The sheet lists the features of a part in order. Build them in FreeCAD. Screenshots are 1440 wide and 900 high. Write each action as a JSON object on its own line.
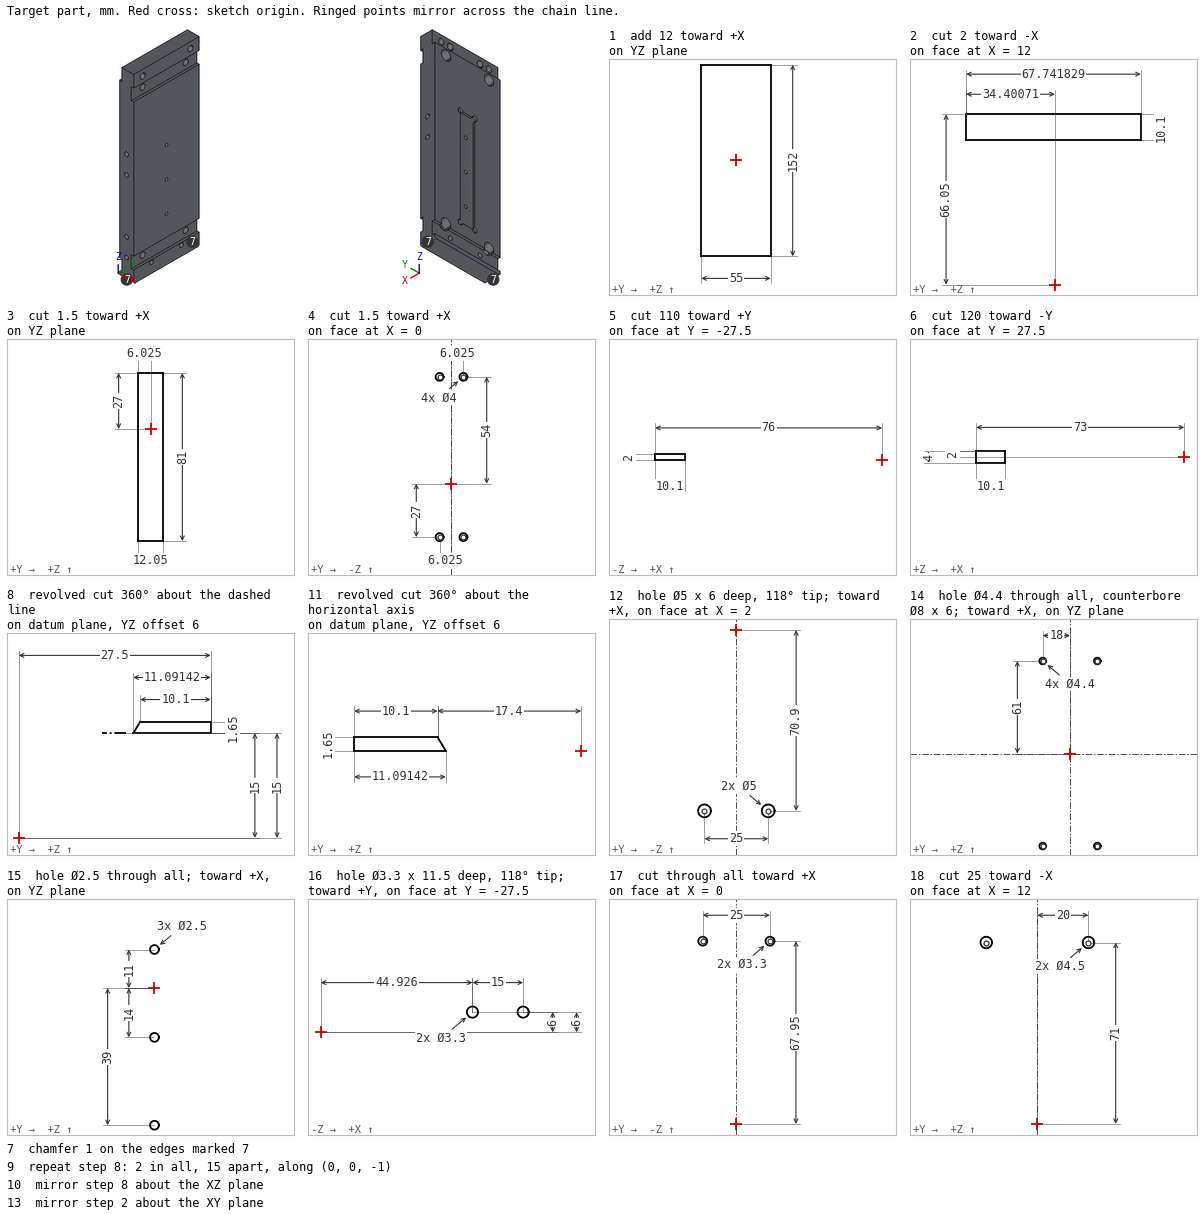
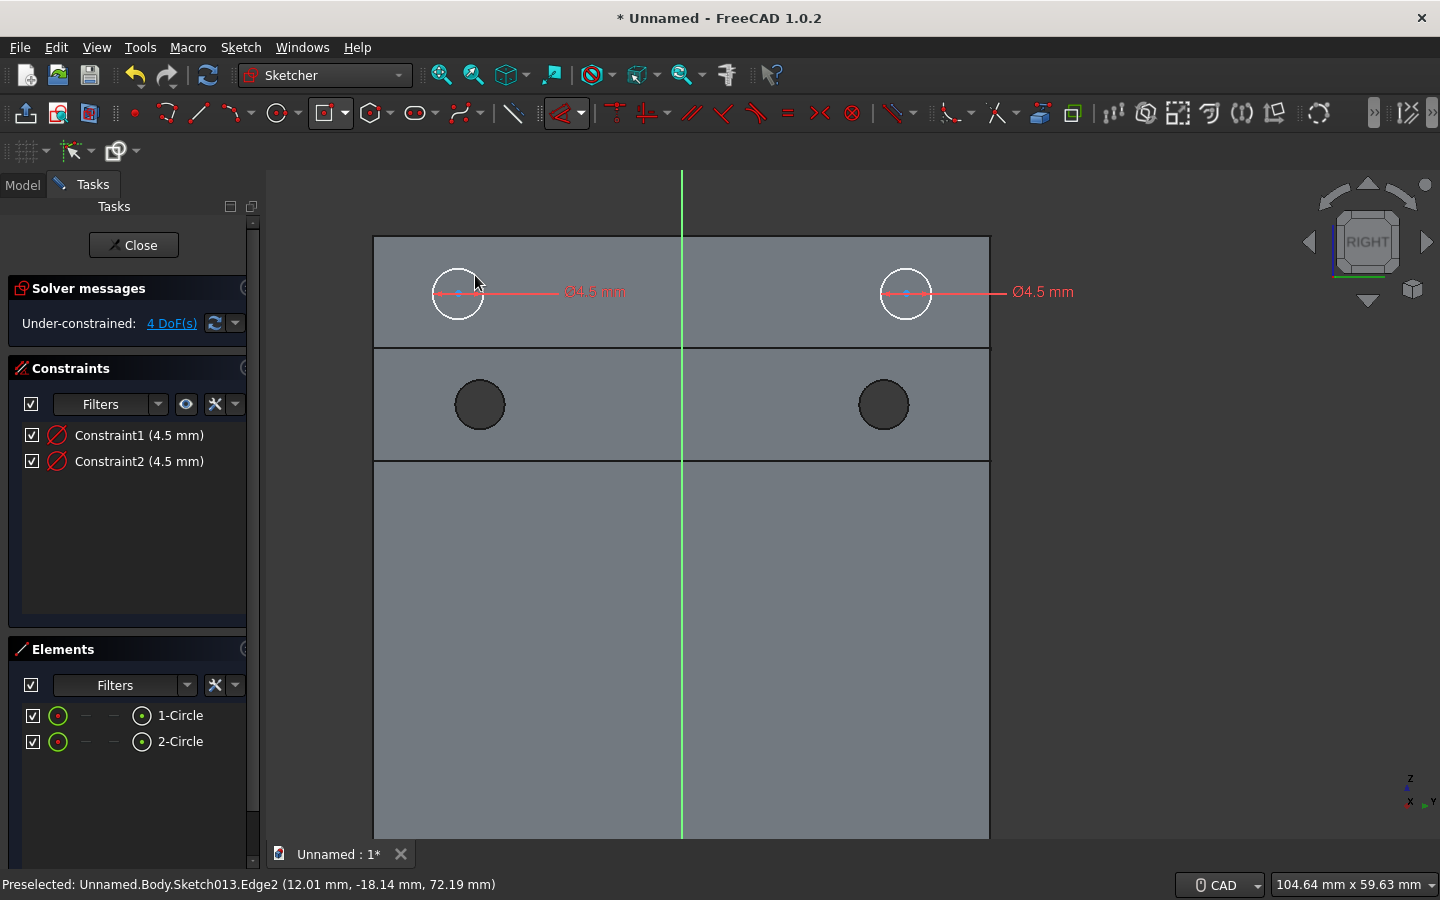
{"action": "left_click", "coordinate": [906, 294]}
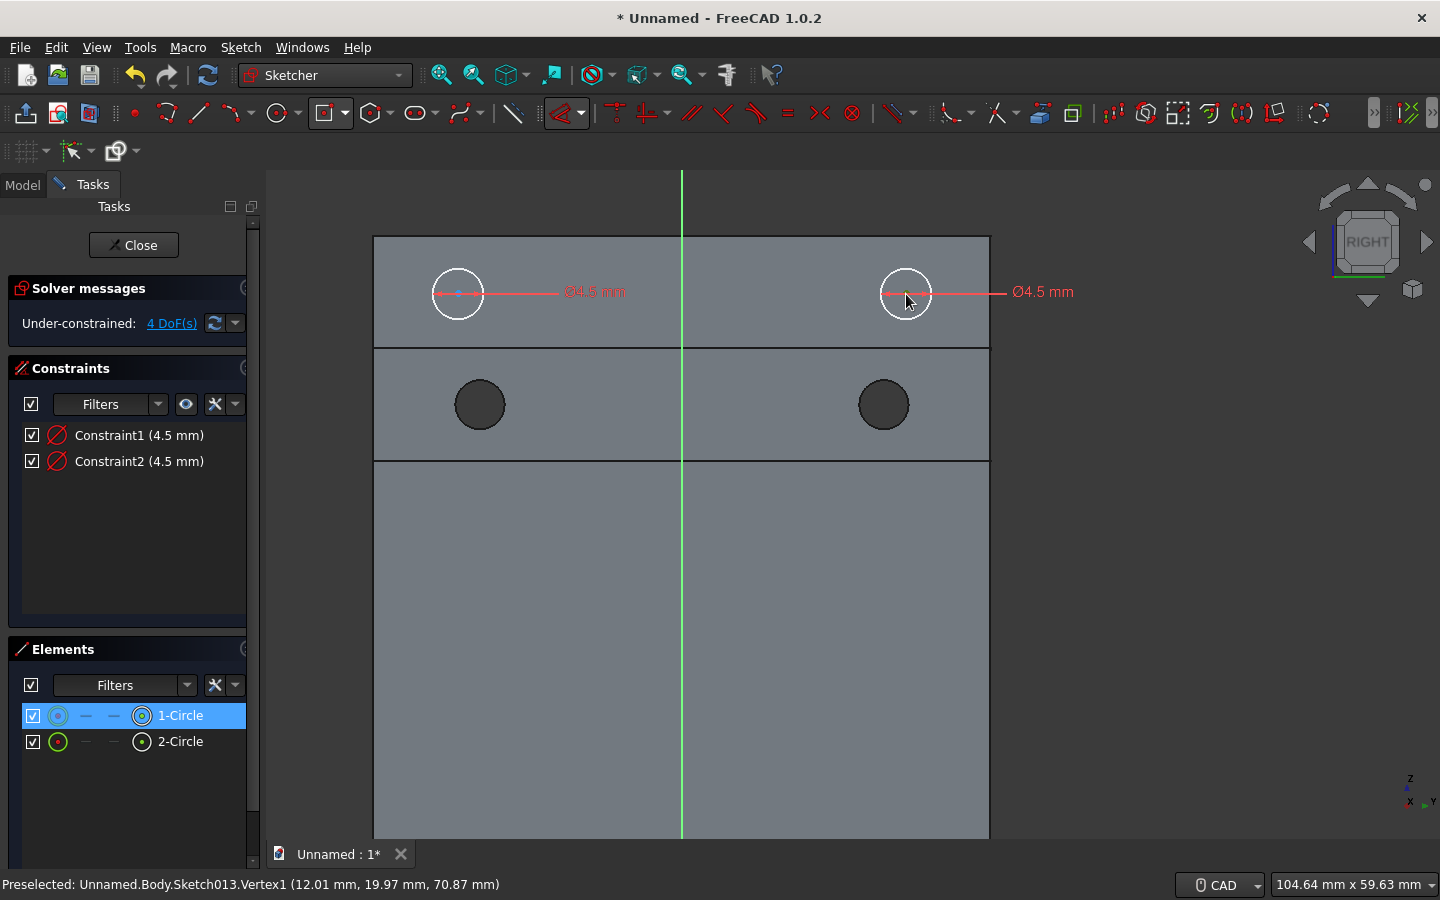
{"action": "left_click", "coordinate": [458, 294]}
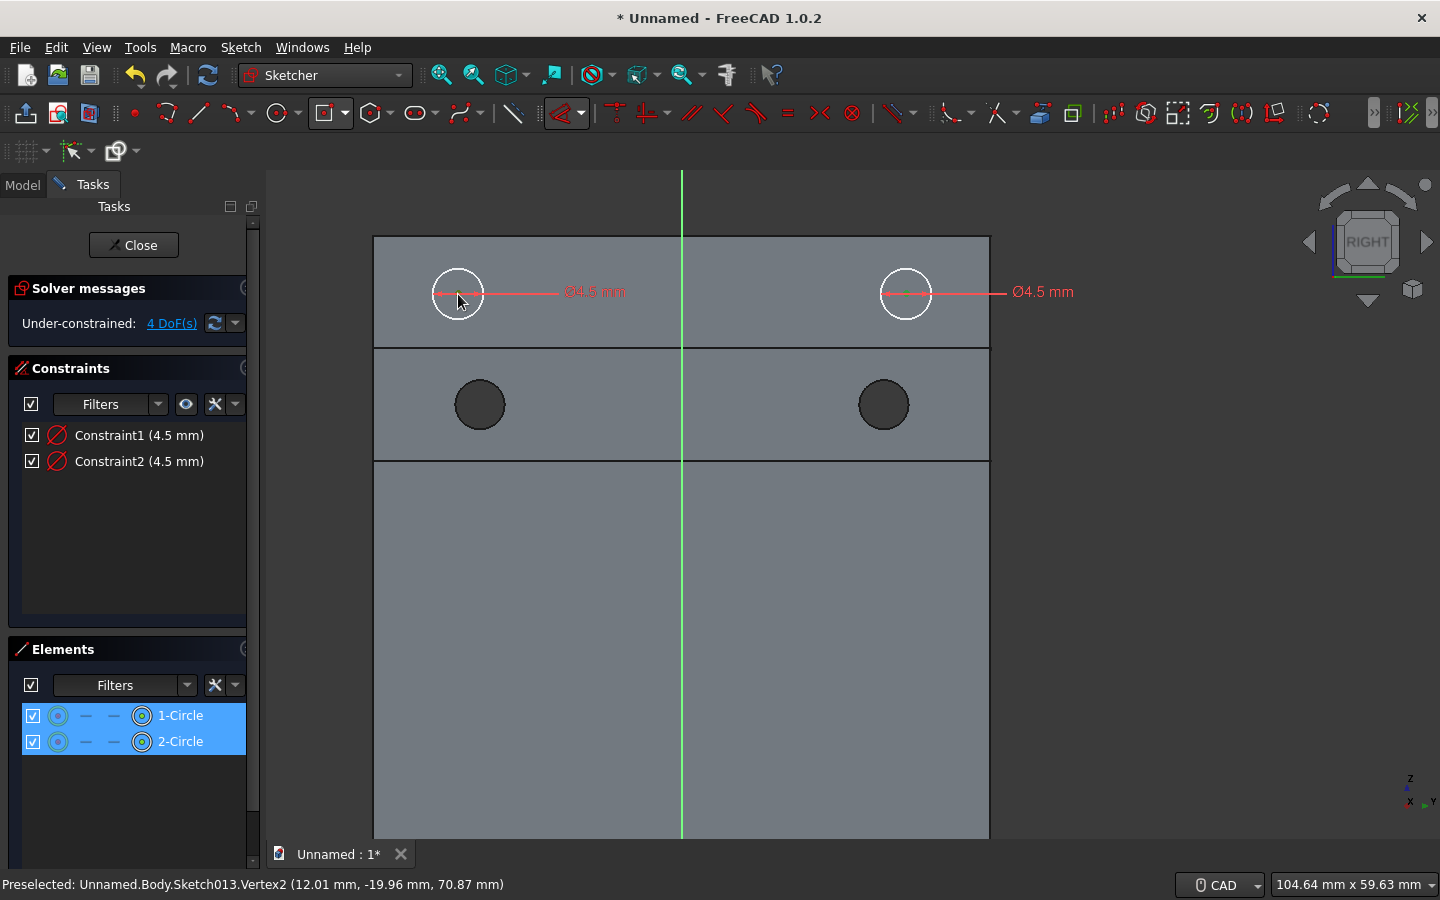
{"action": "left_click", "coordinate": [682, 767]}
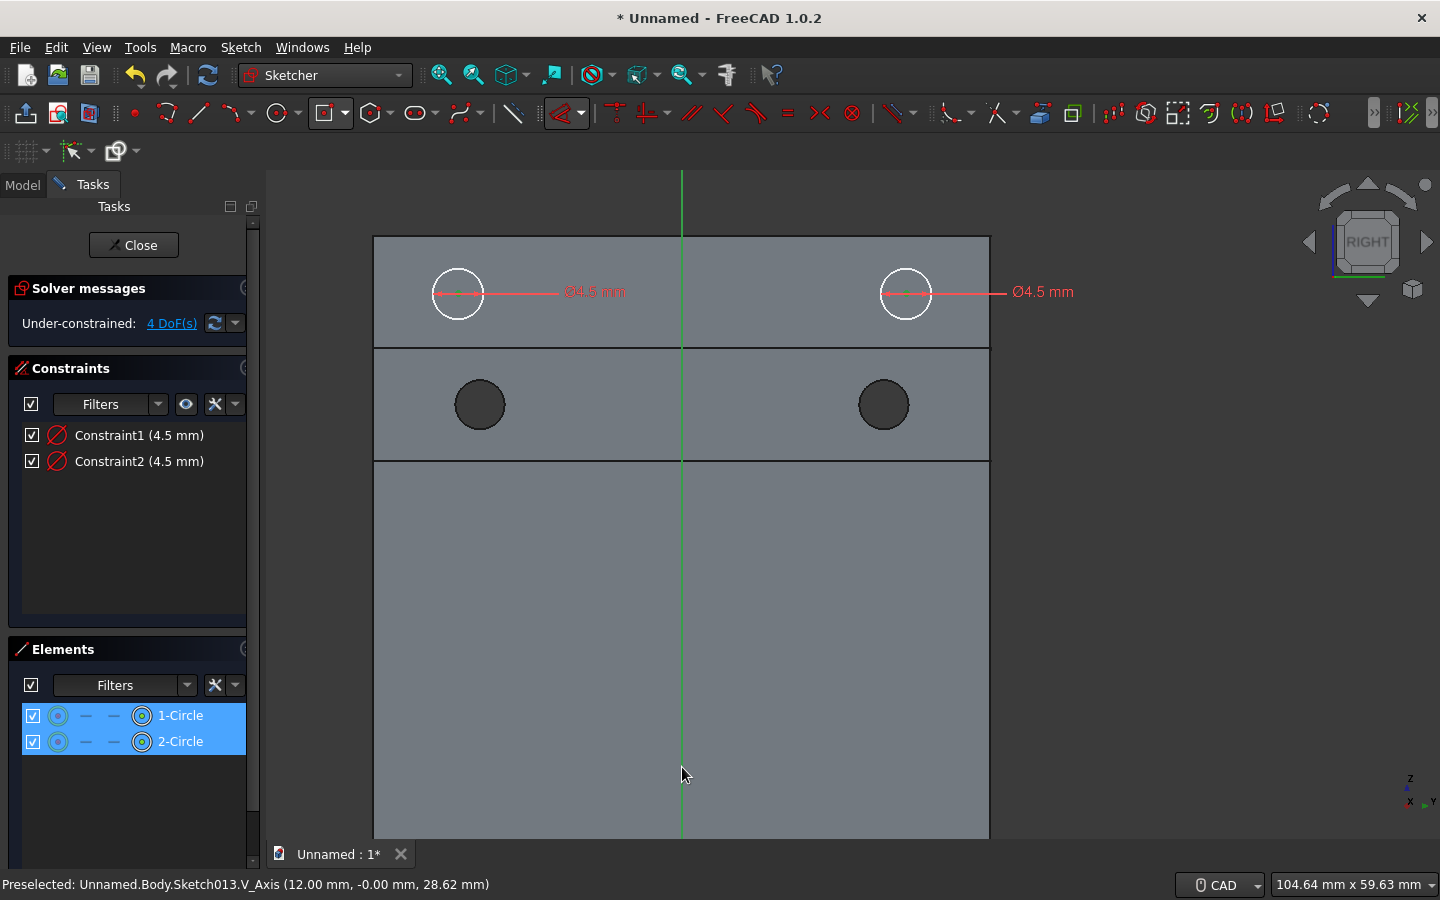
{"action": "left_click", "coordinate": [820, 114]}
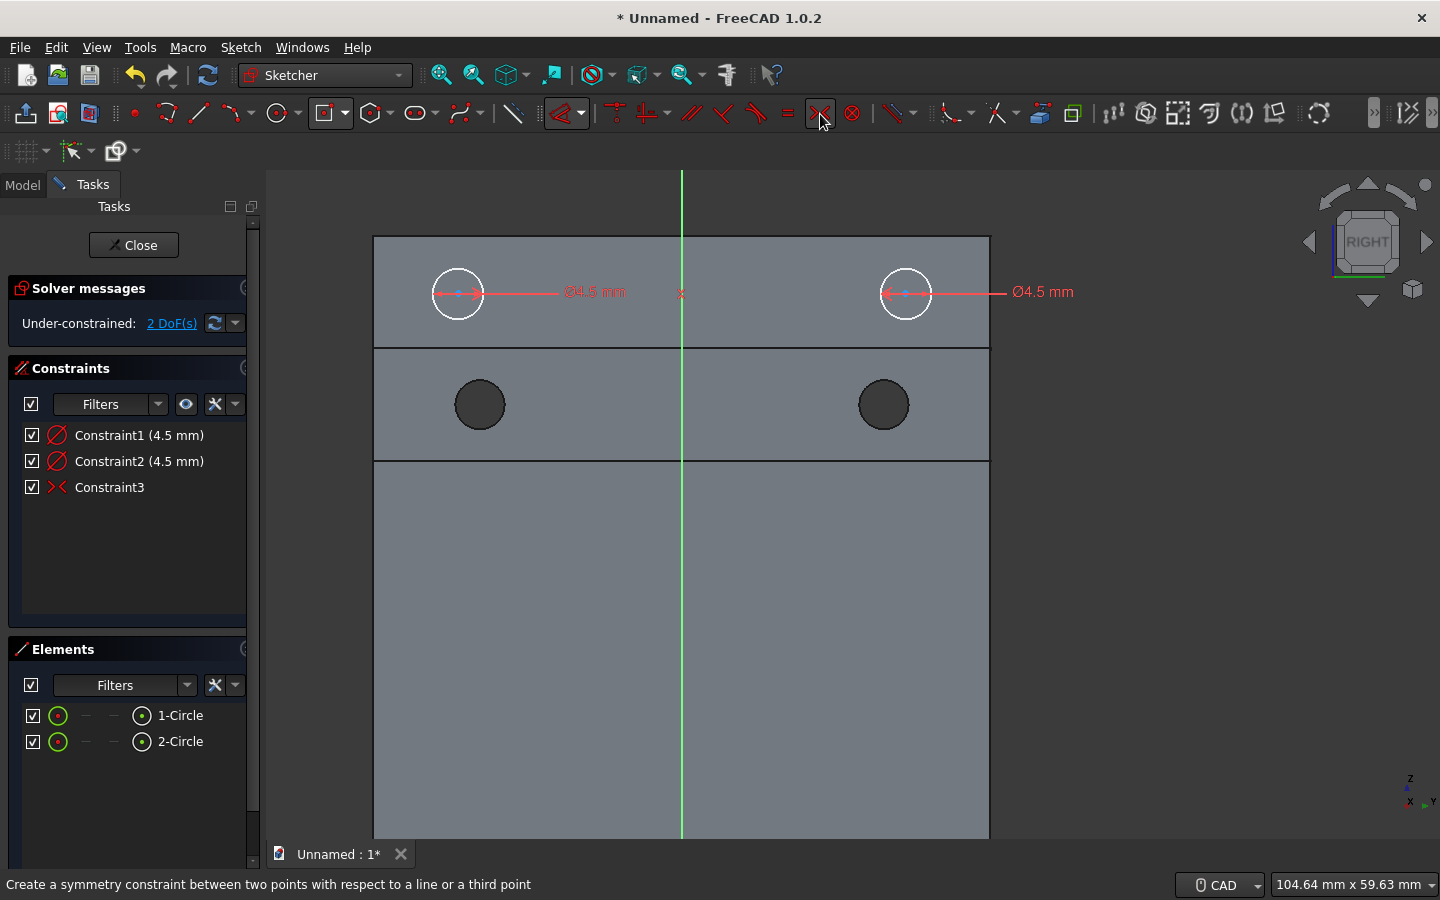
{"action": "left_click", "coordinate": [906, 294]}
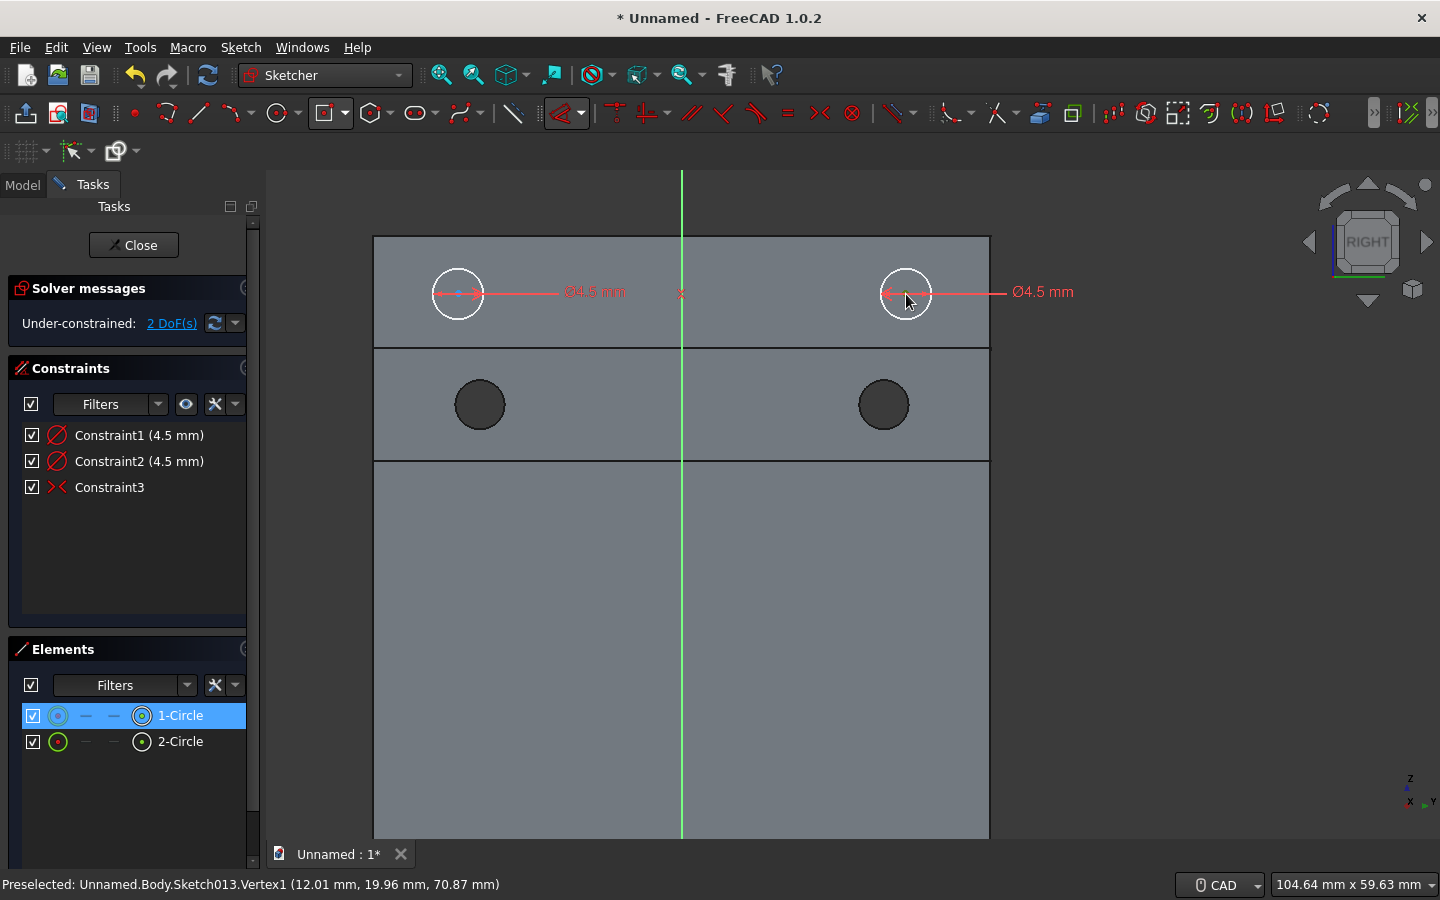
{"action": "left_click", "coordinate": [584, 114]}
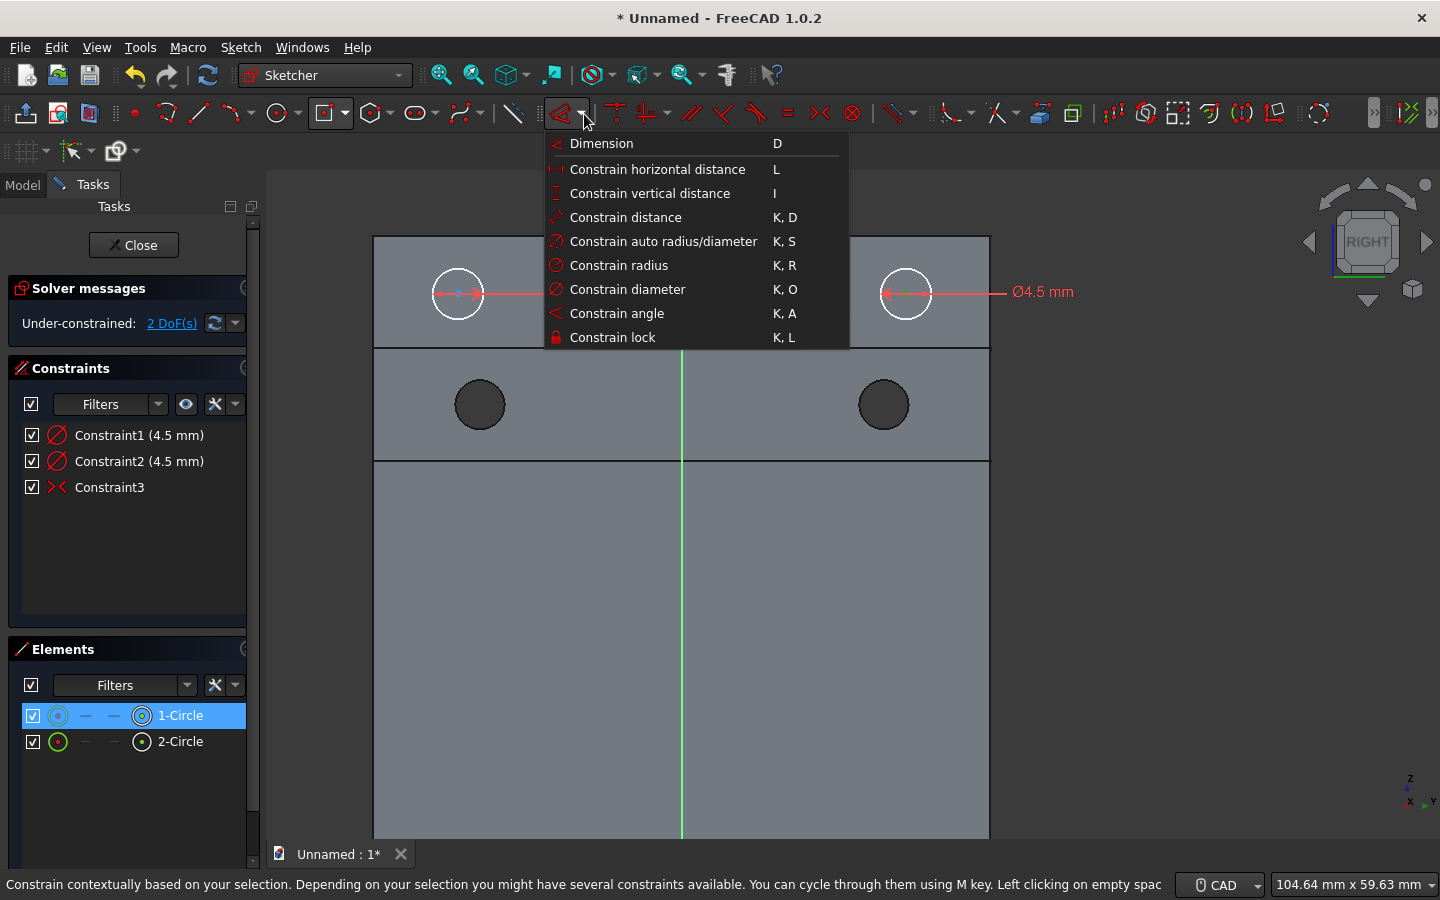
{"action": "left_click", "coordinate": [697, 169]}